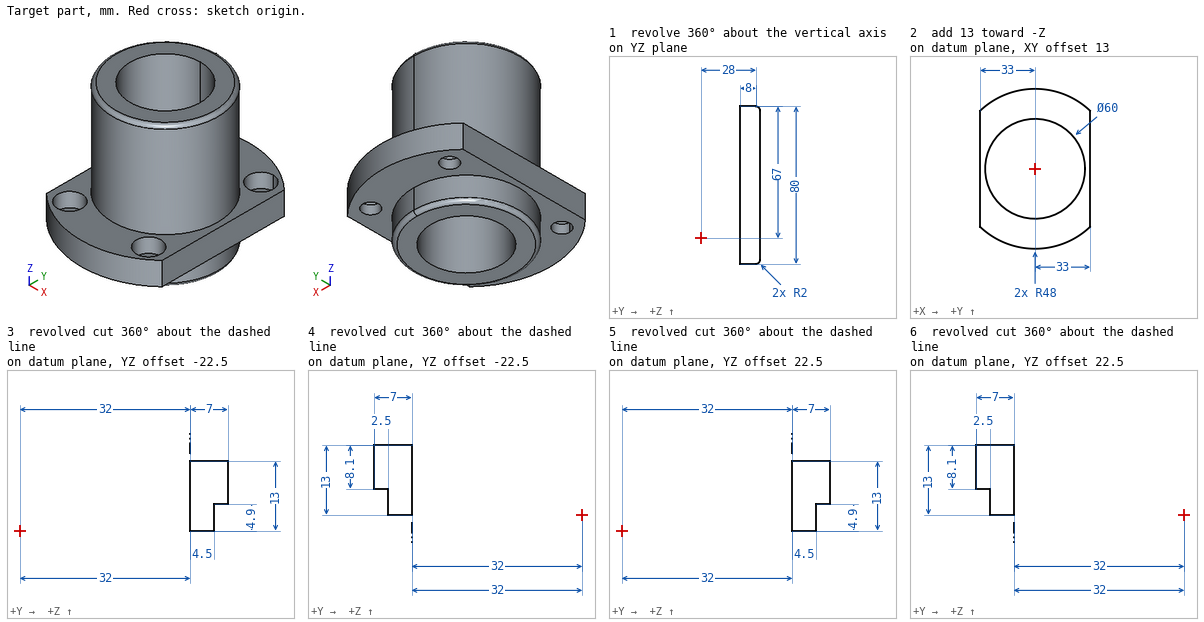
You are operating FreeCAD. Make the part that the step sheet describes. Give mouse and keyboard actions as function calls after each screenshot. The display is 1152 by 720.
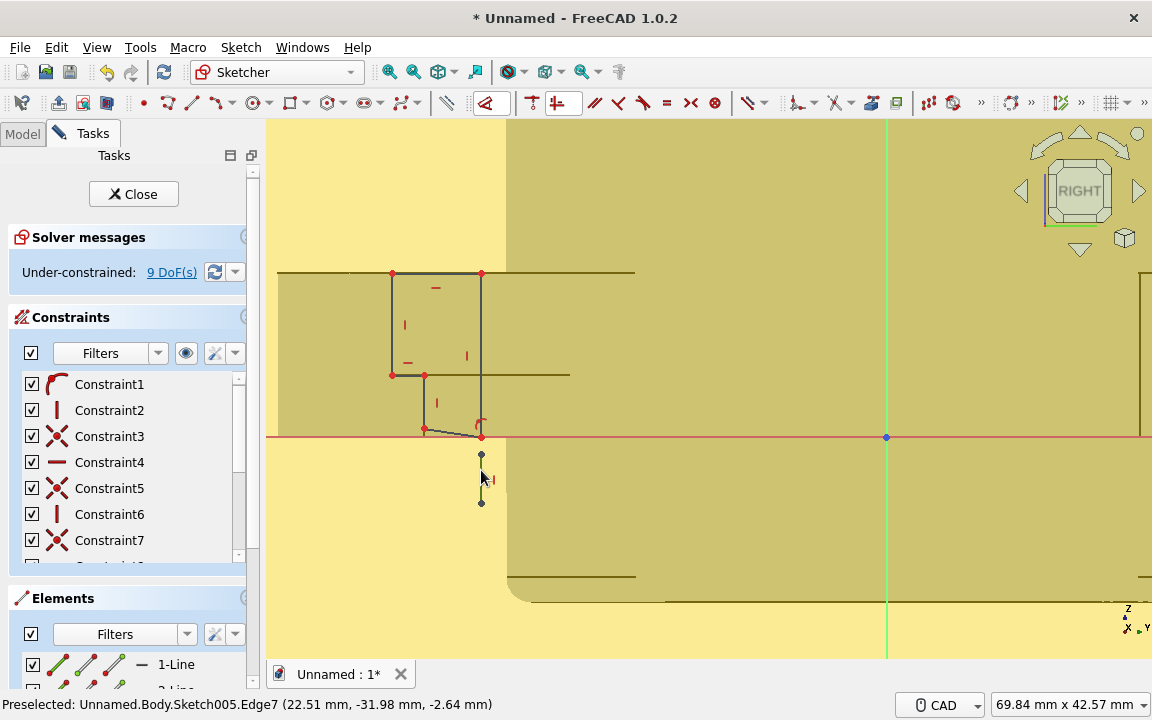
click(448, 104)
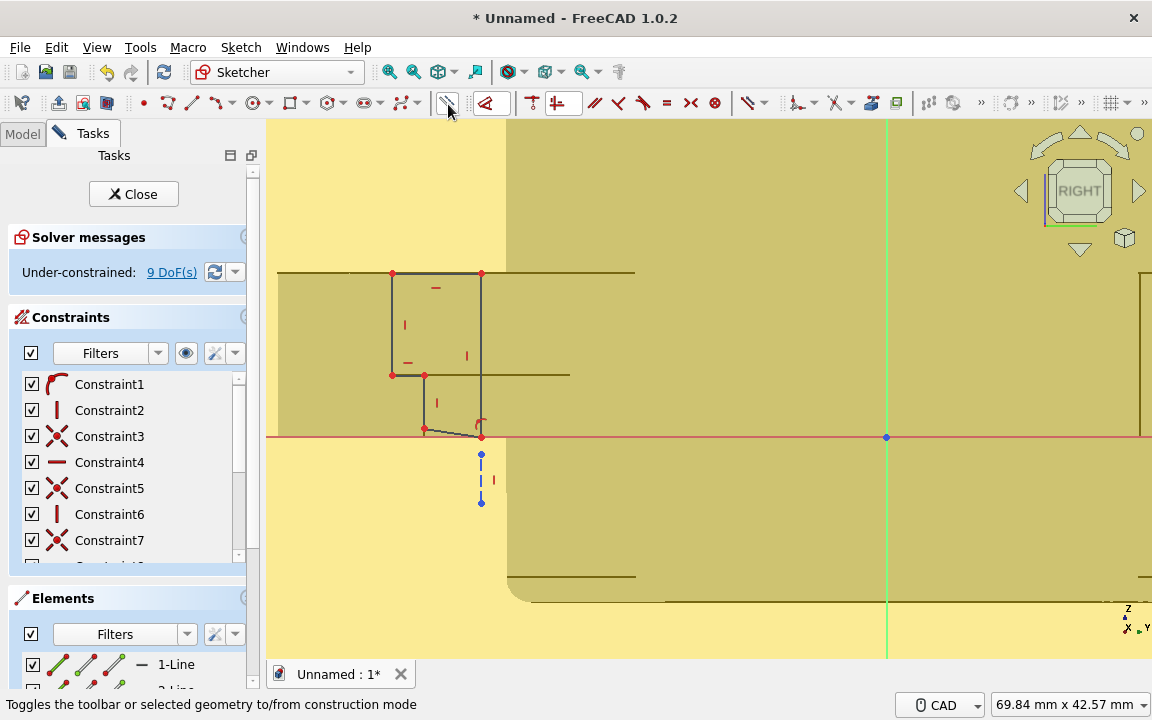
click(464, 435)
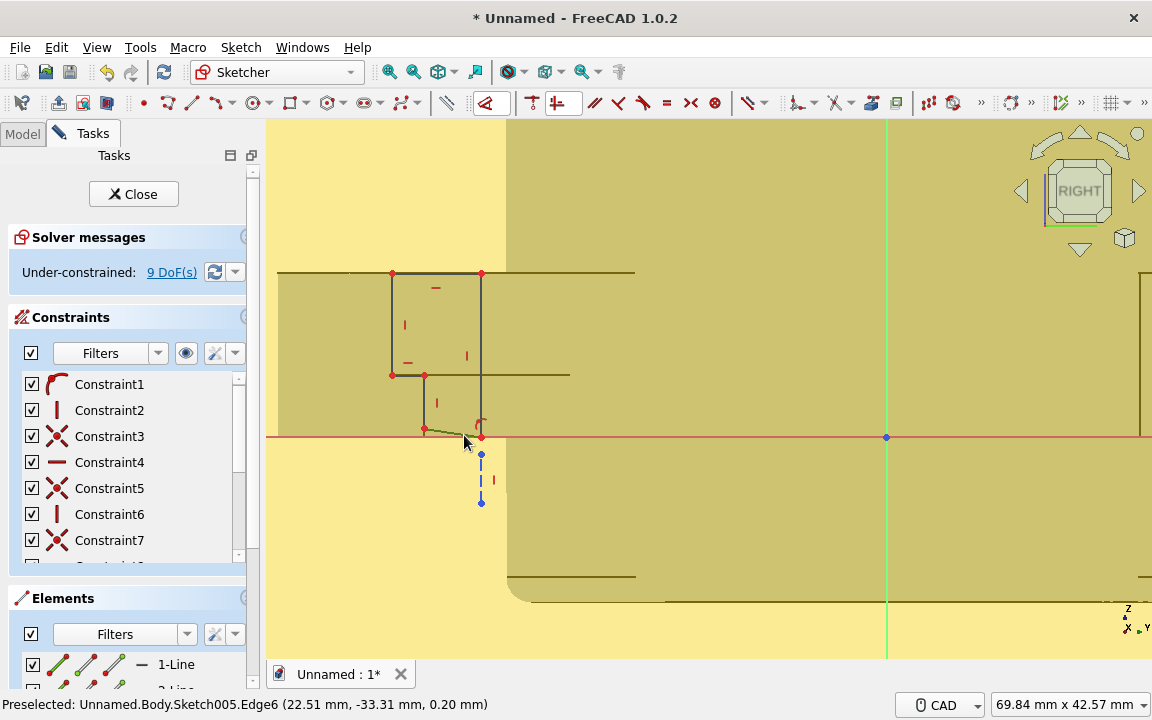
click(576, 104)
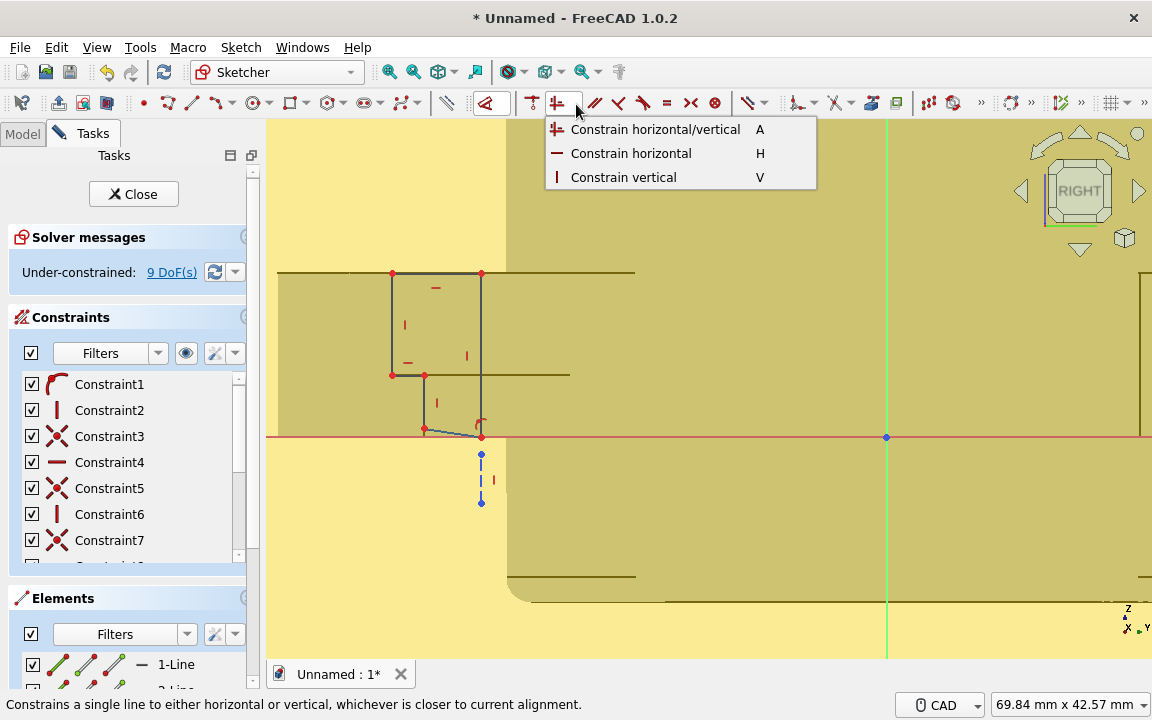
click(681, 153)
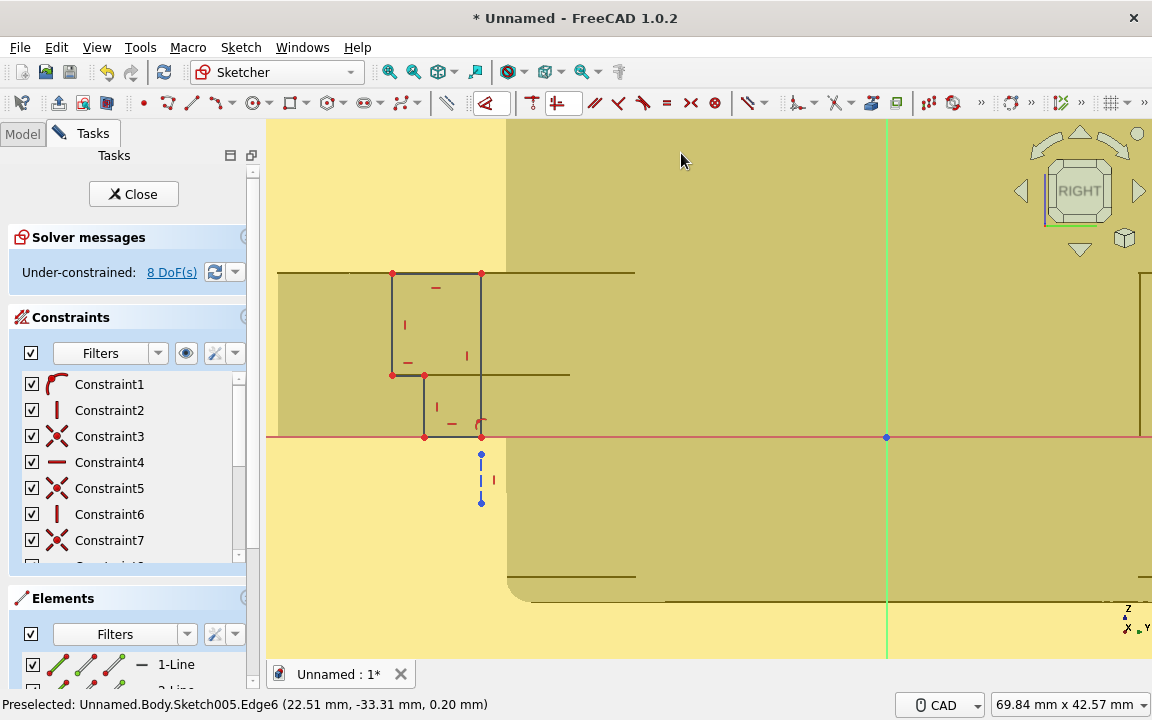
click(454, 274)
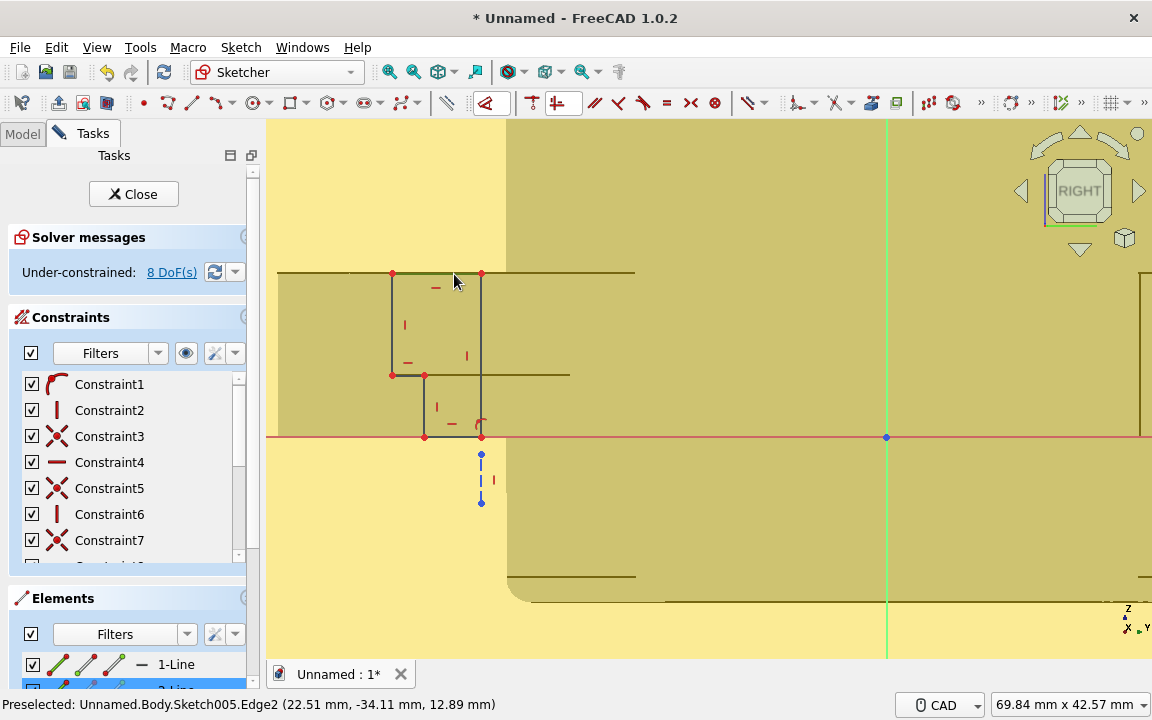
key(l)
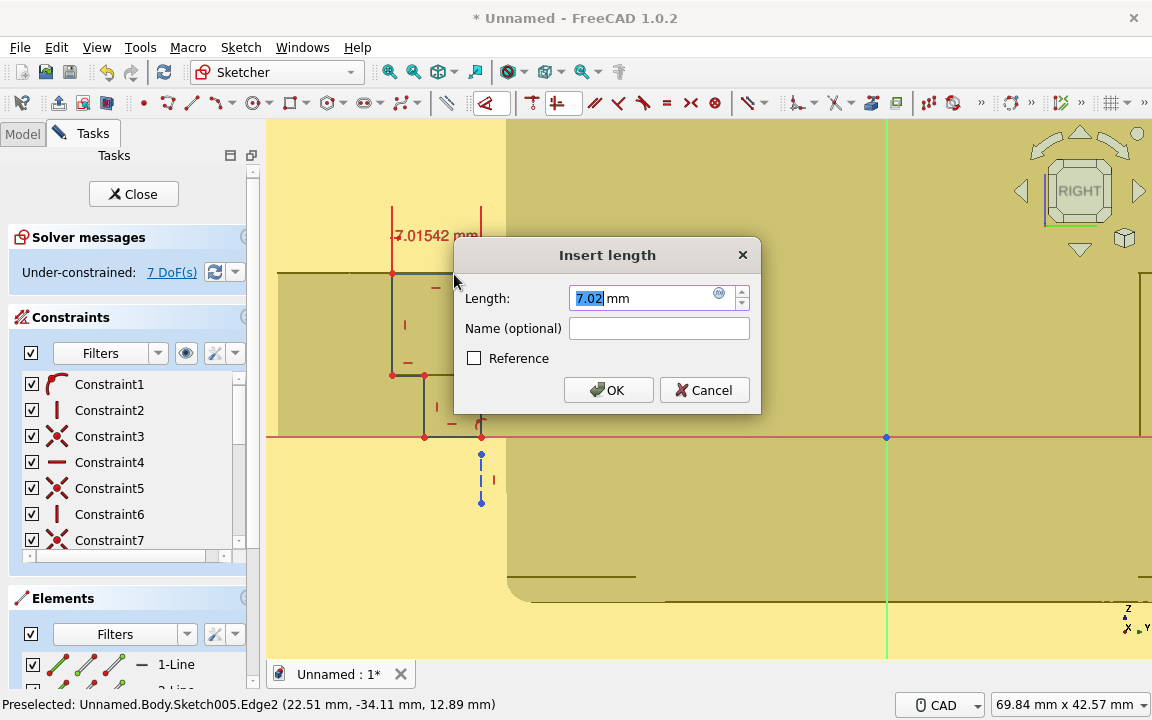
text(7)
key(Return)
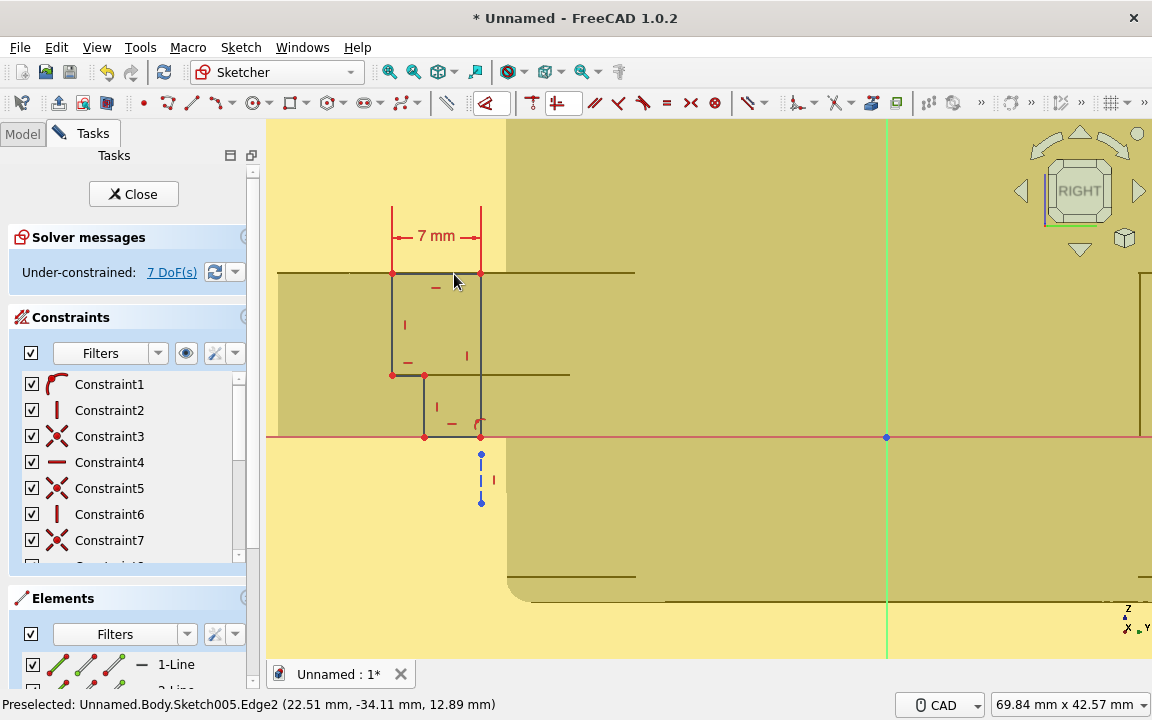
click(481, 388)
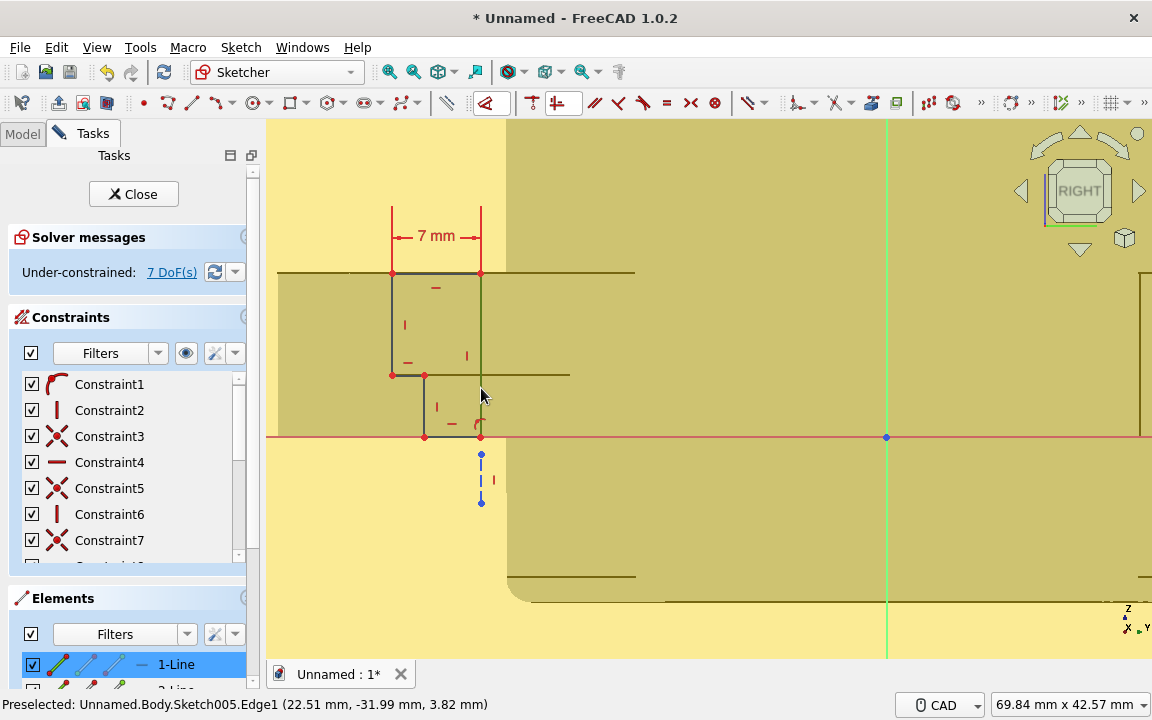
click(504, 104)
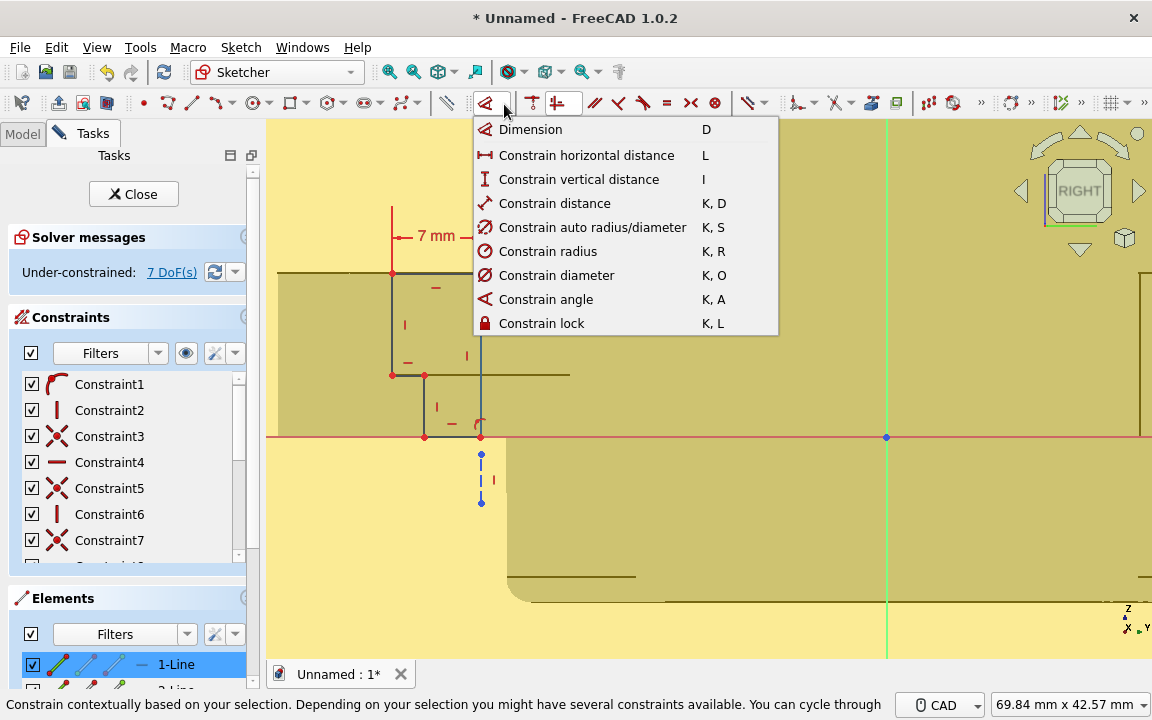
click(626, 179)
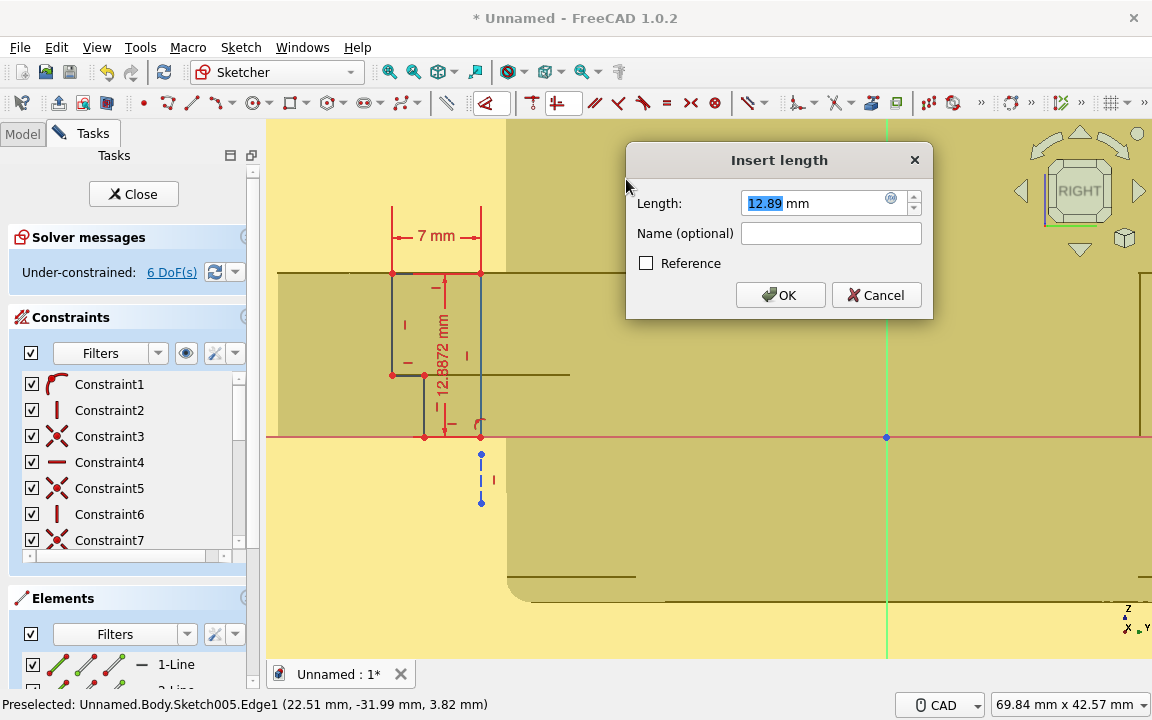
text(13)
key(Return)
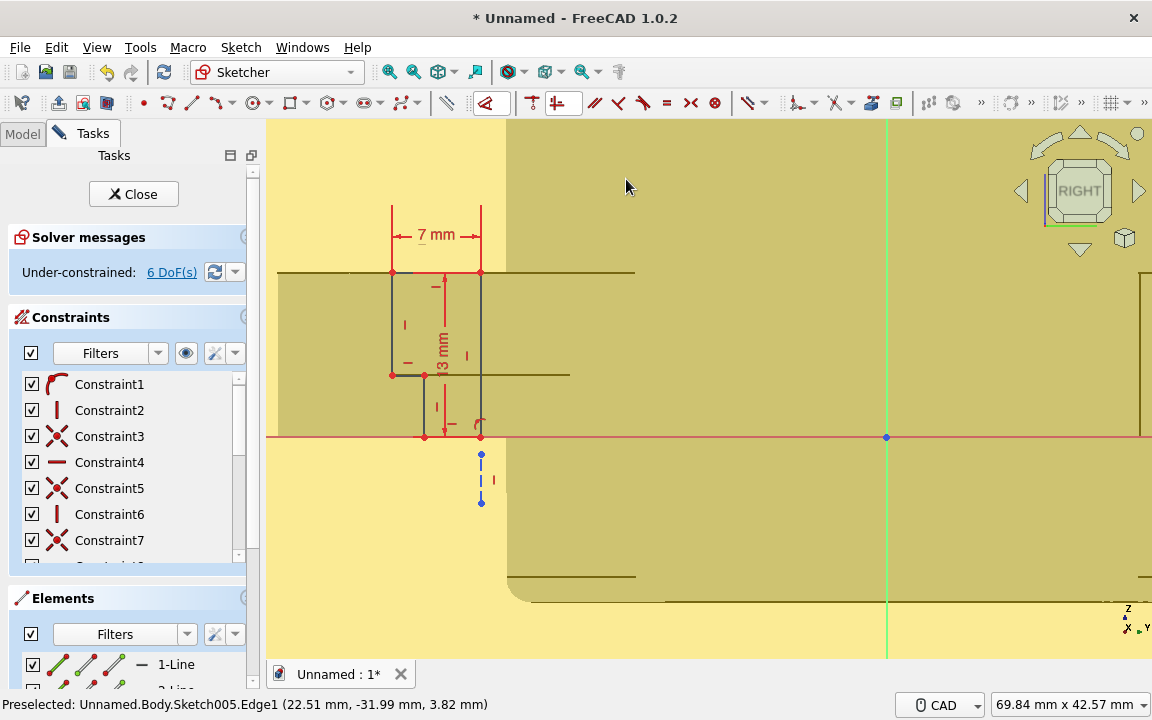
click(392, 304)